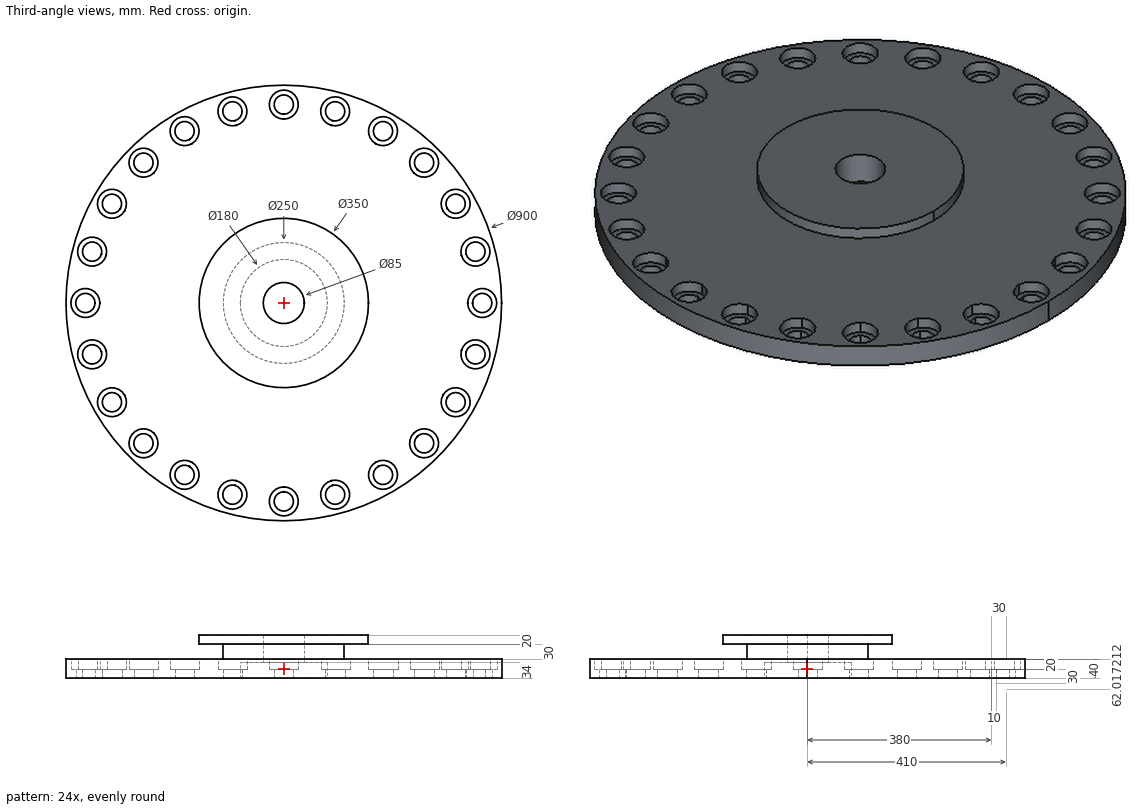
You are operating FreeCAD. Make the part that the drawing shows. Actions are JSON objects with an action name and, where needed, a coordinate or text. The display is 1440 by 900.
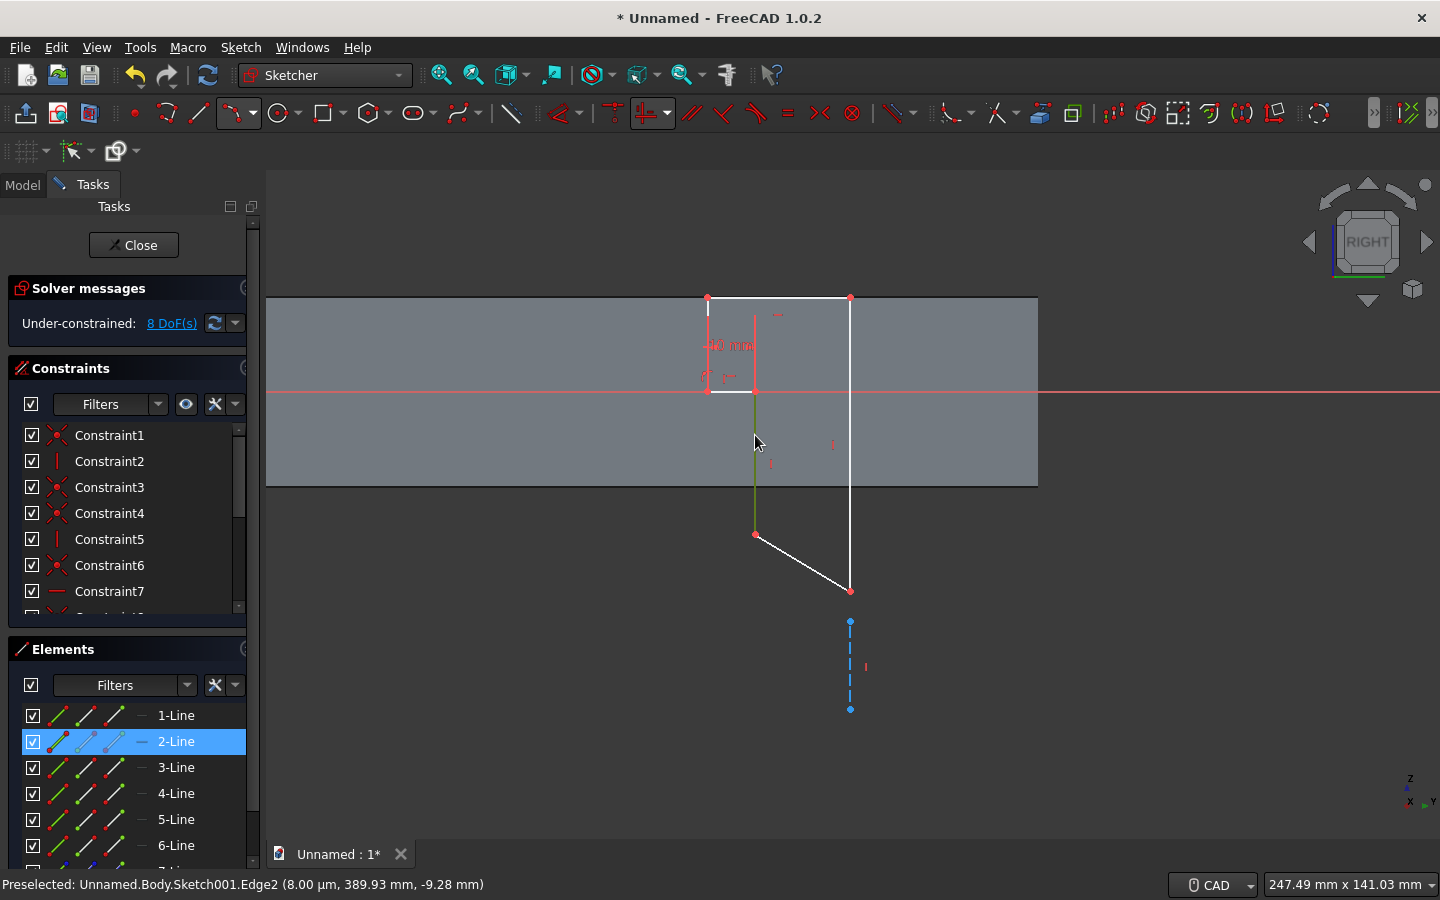
{"action": "key", "text": "i"}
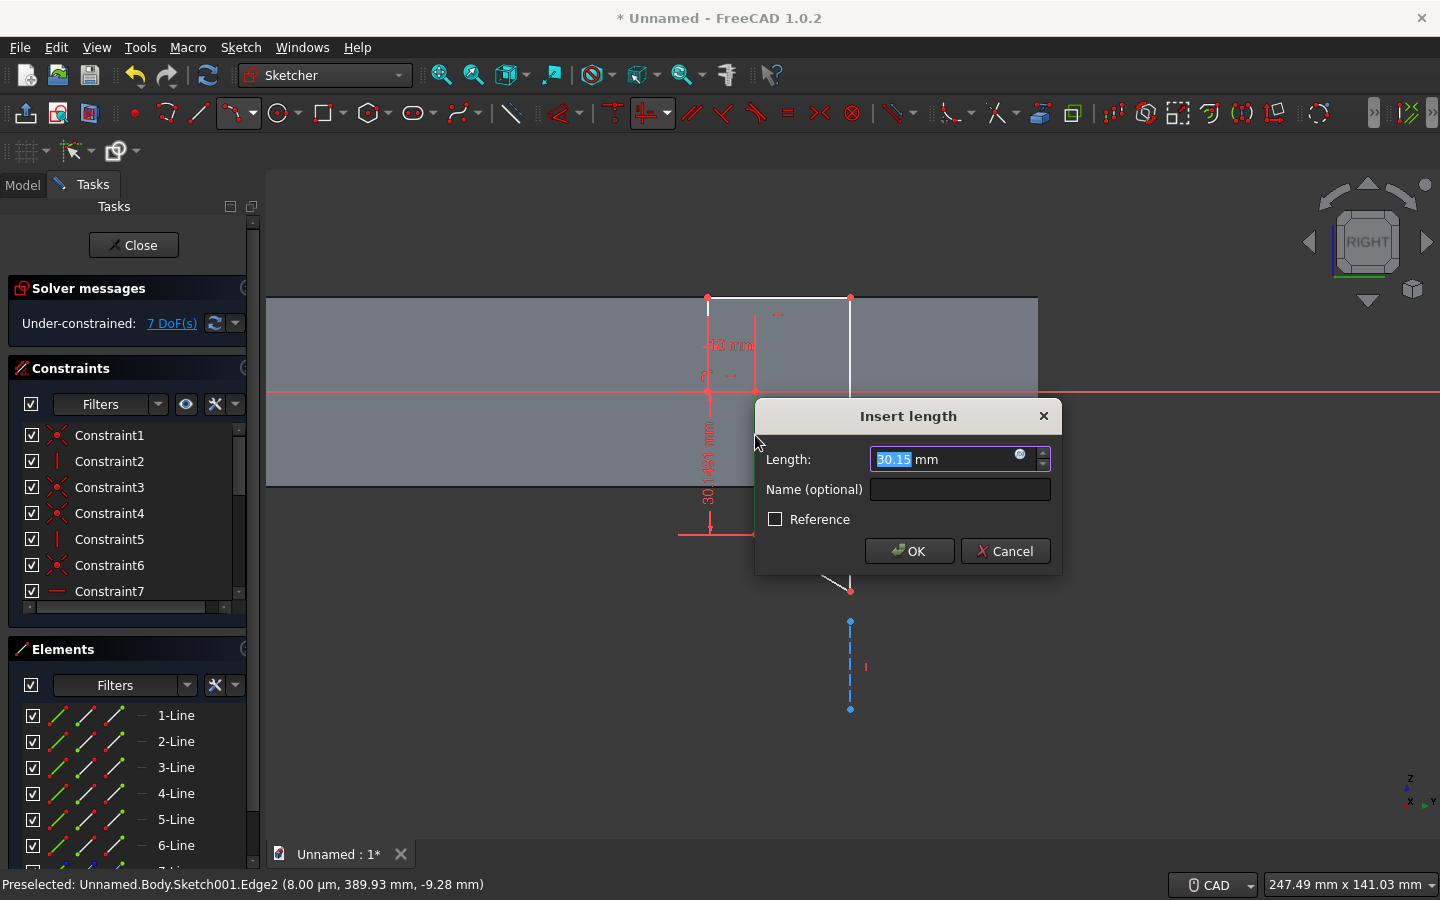
{"action": "type", "text": "30"}
{"action": "key", "text": "Return"}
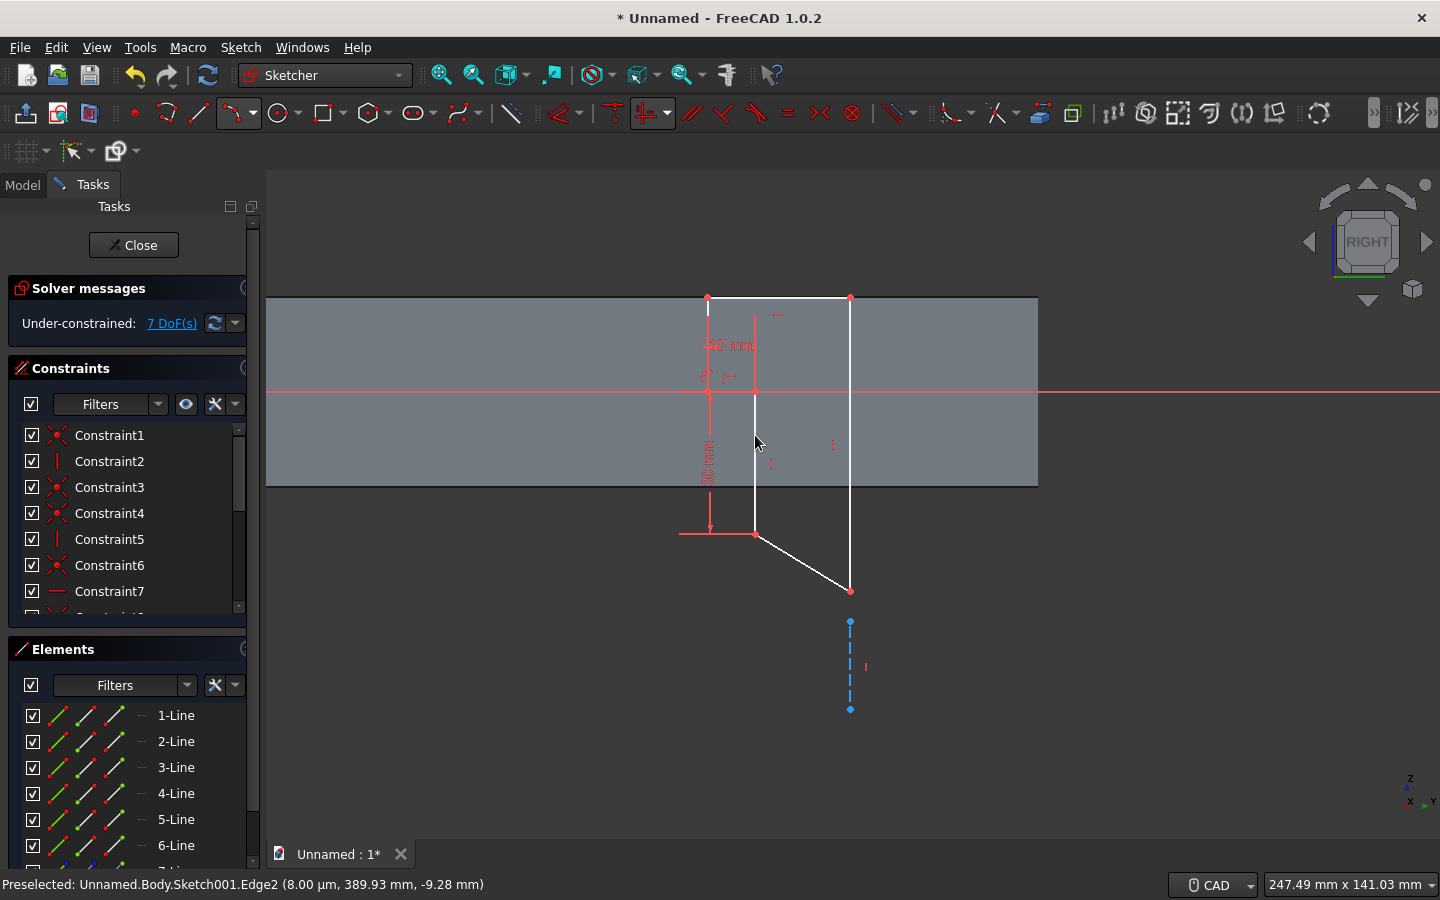
{"action": "left_click", "coordinate": [807, 298]}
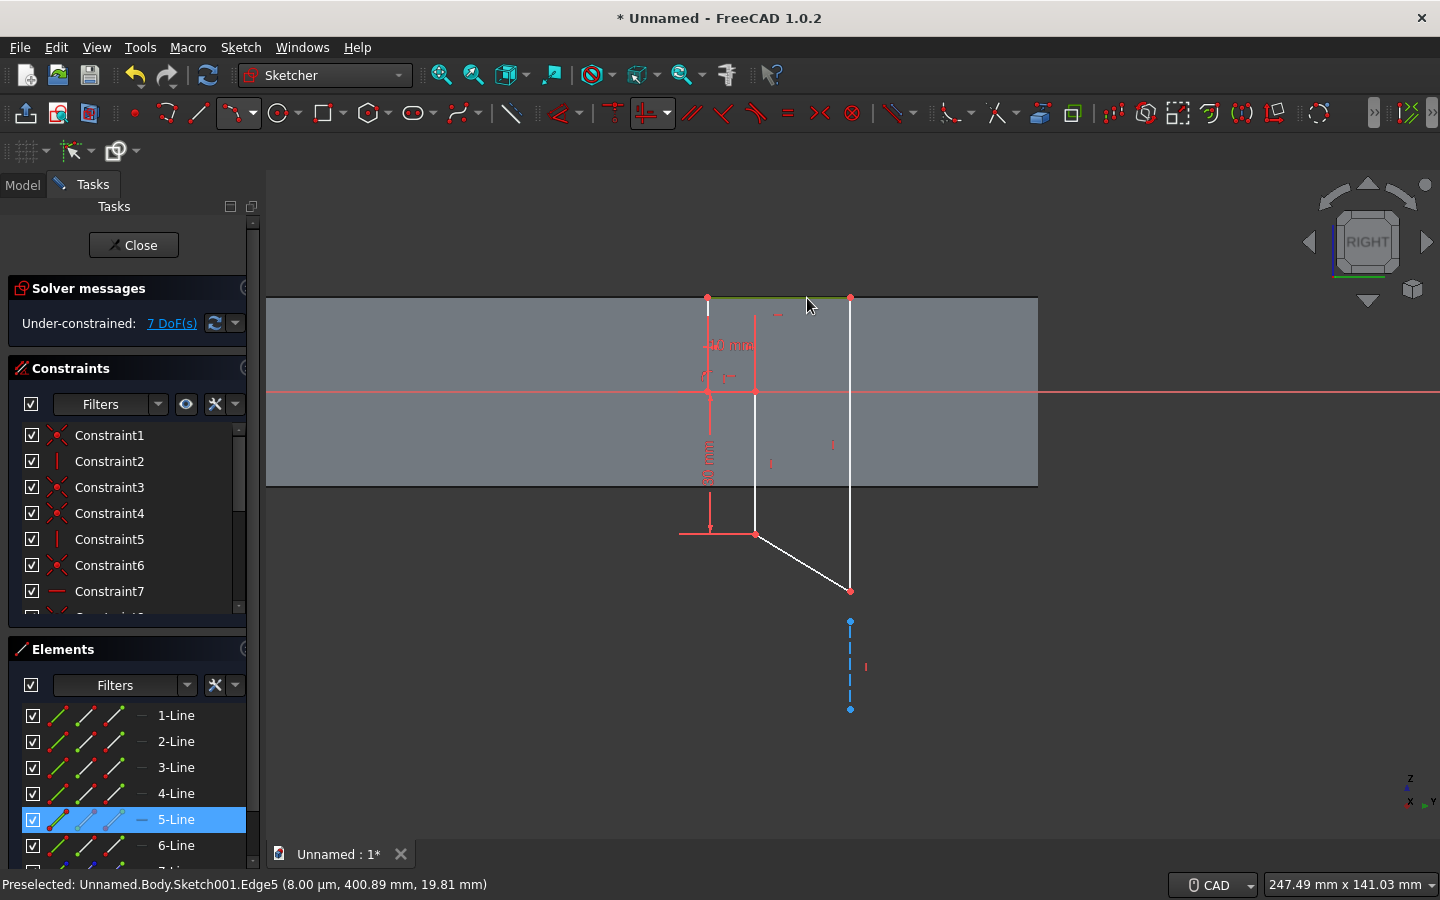
{"action": "key", "text": "l"}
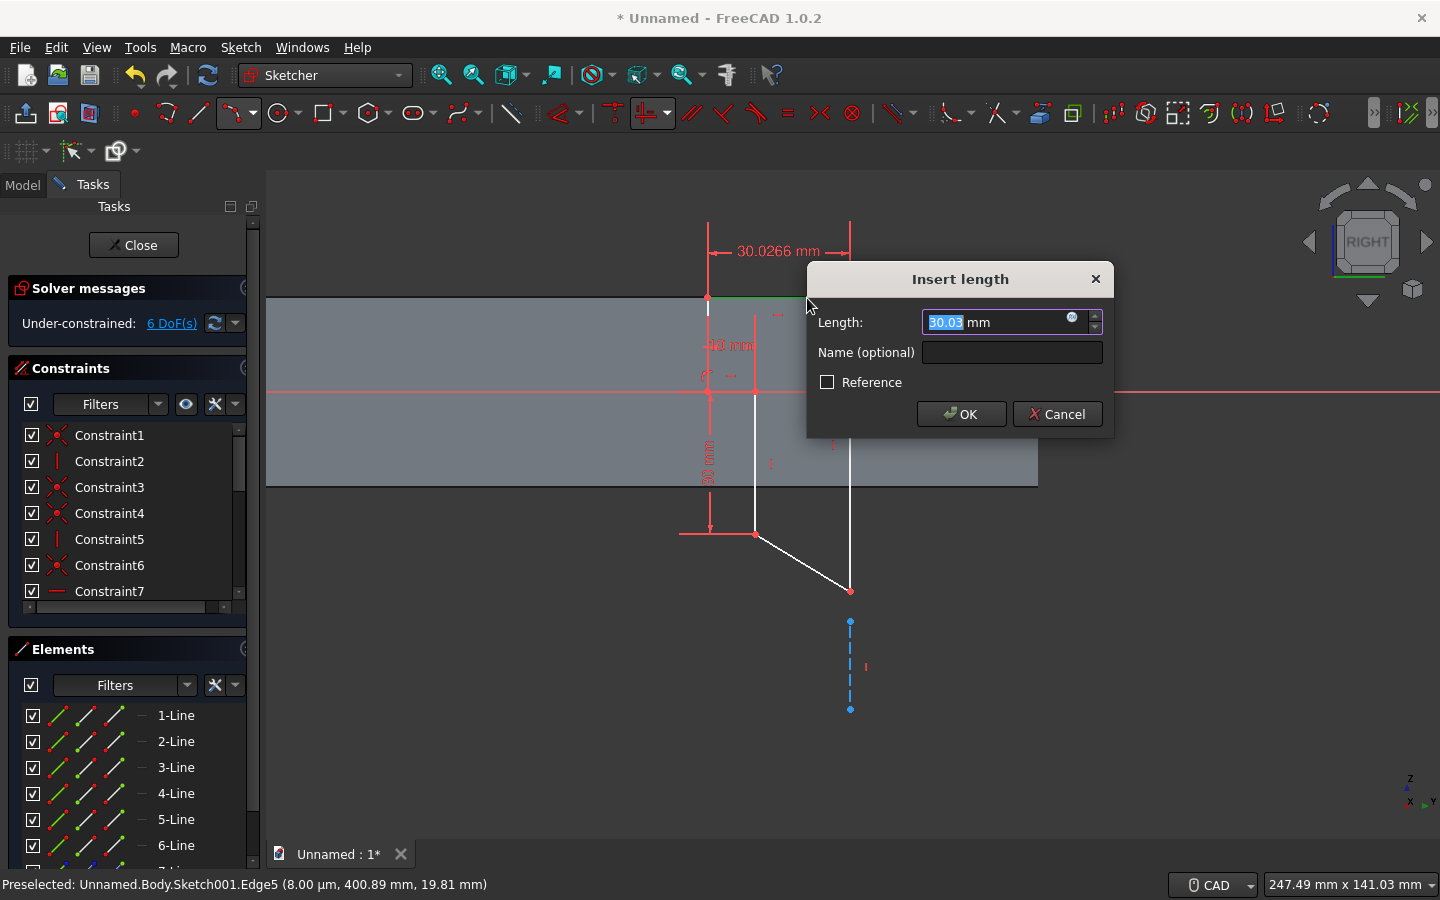
{"action": "type", "text": "30"}
{"action": "key", "text": "Return"}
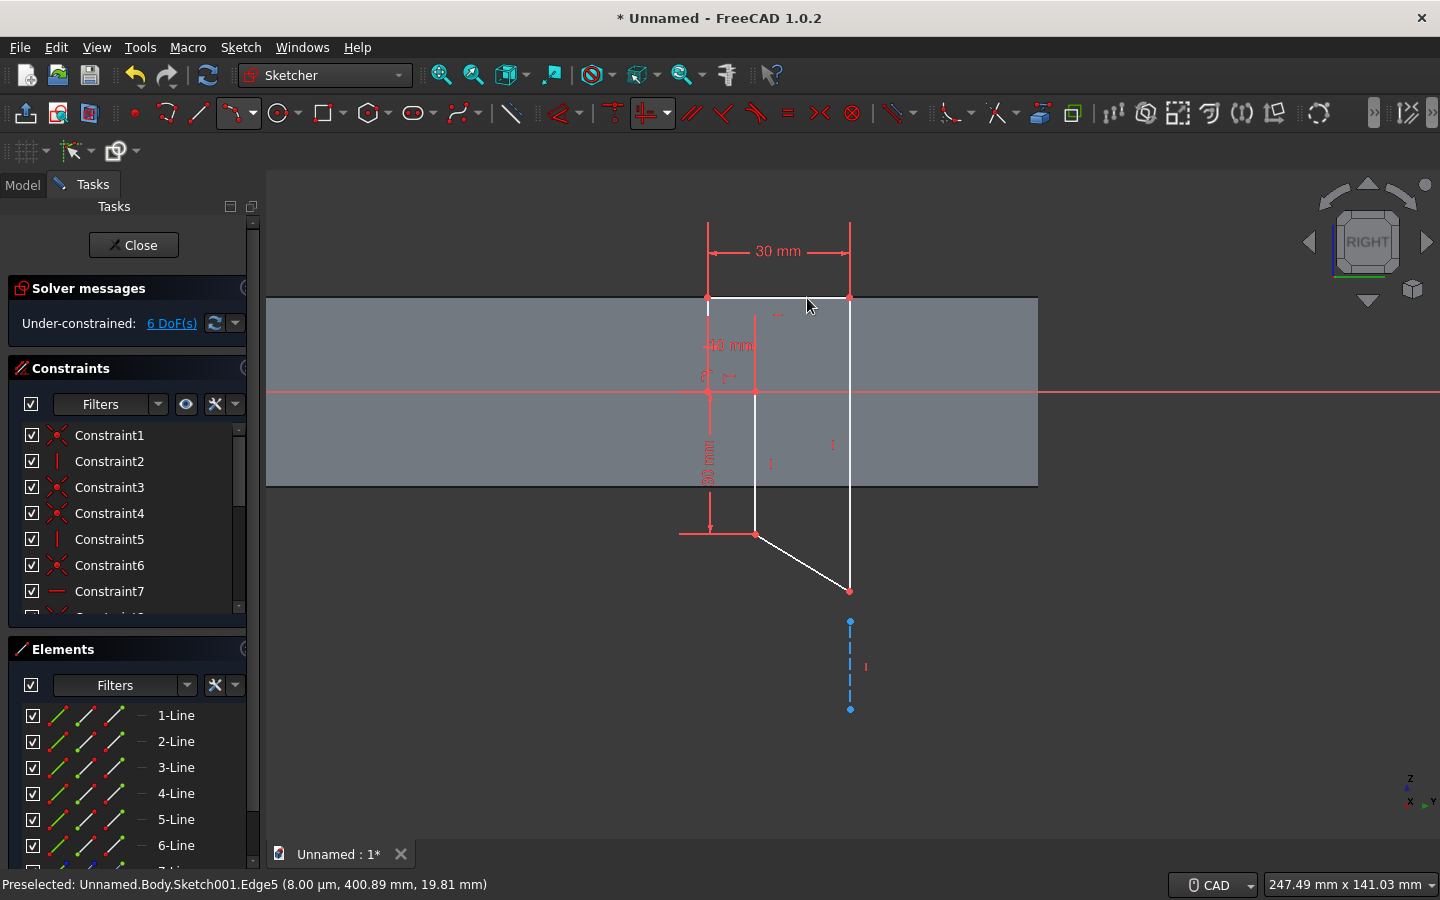
{"action": "left_click", "coordinate": [708, 326]}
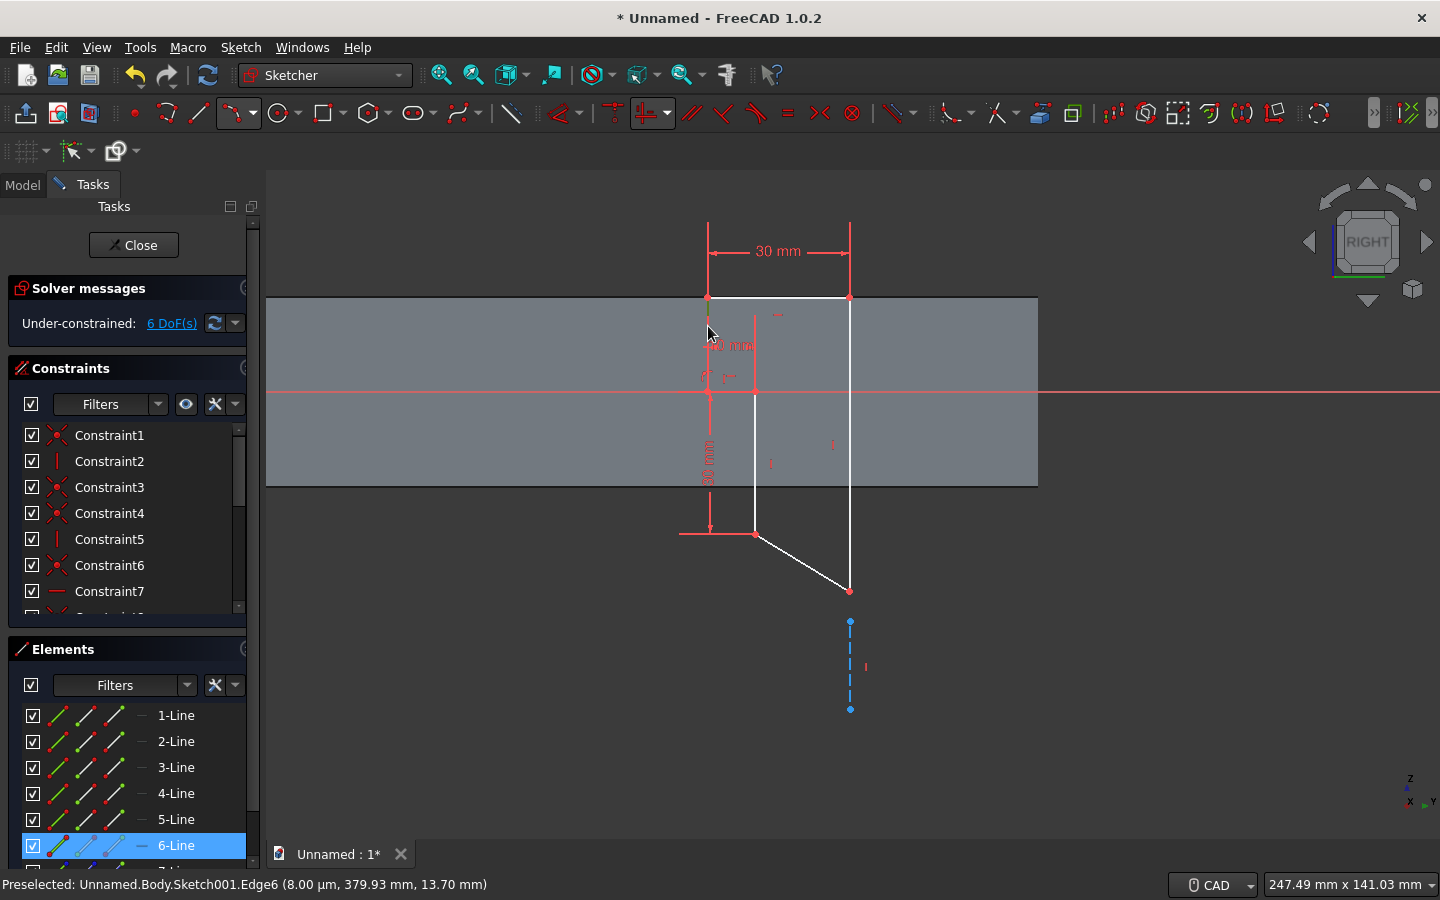
{"action": "key", "text": "i"}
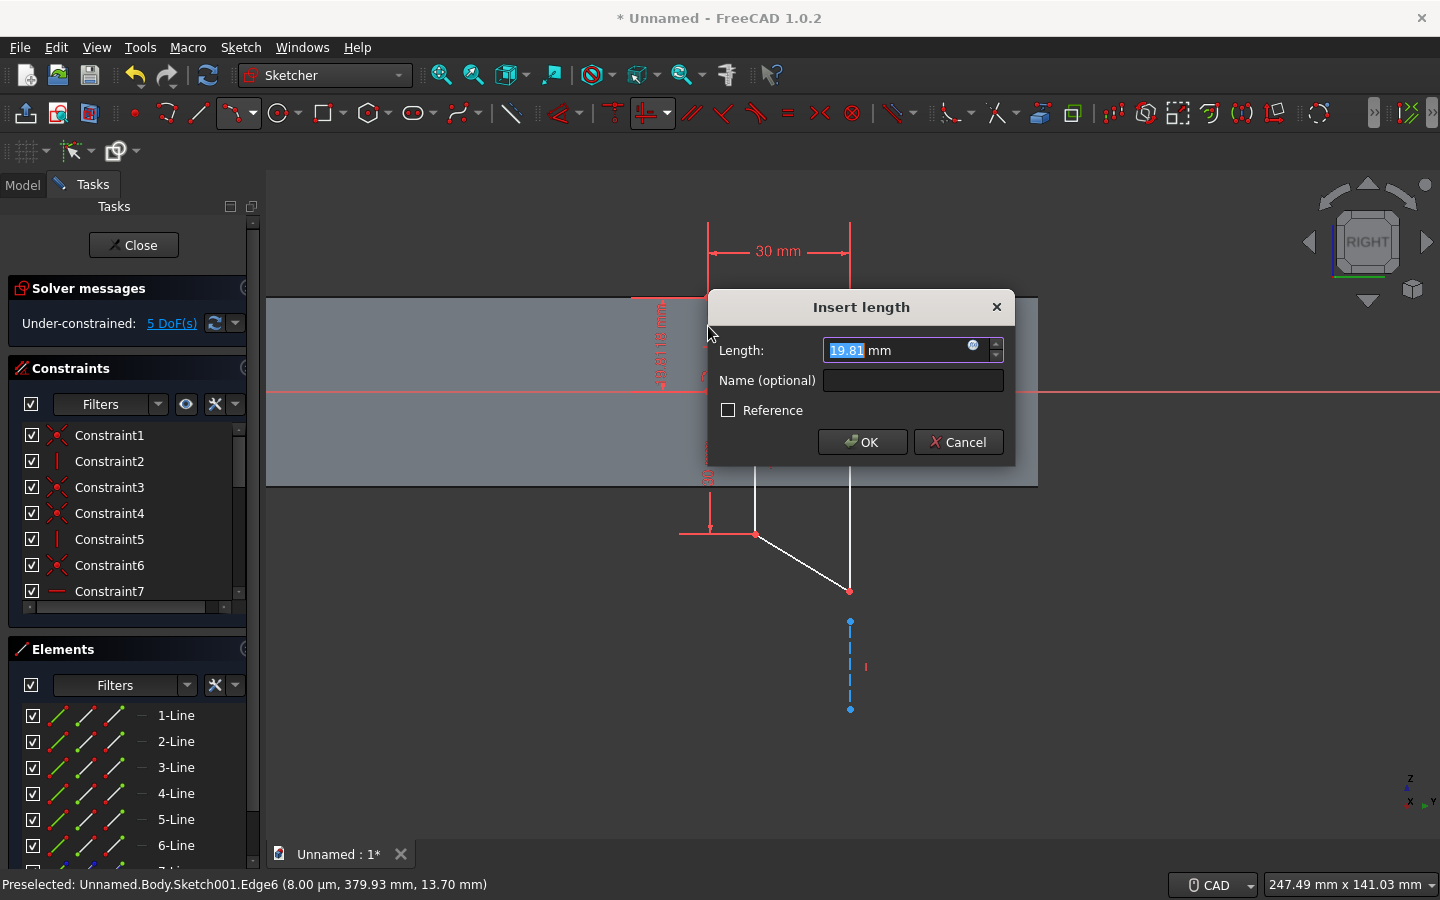
{"action": "type", "text": "20"}
{"action": "key", "text": "Return"}